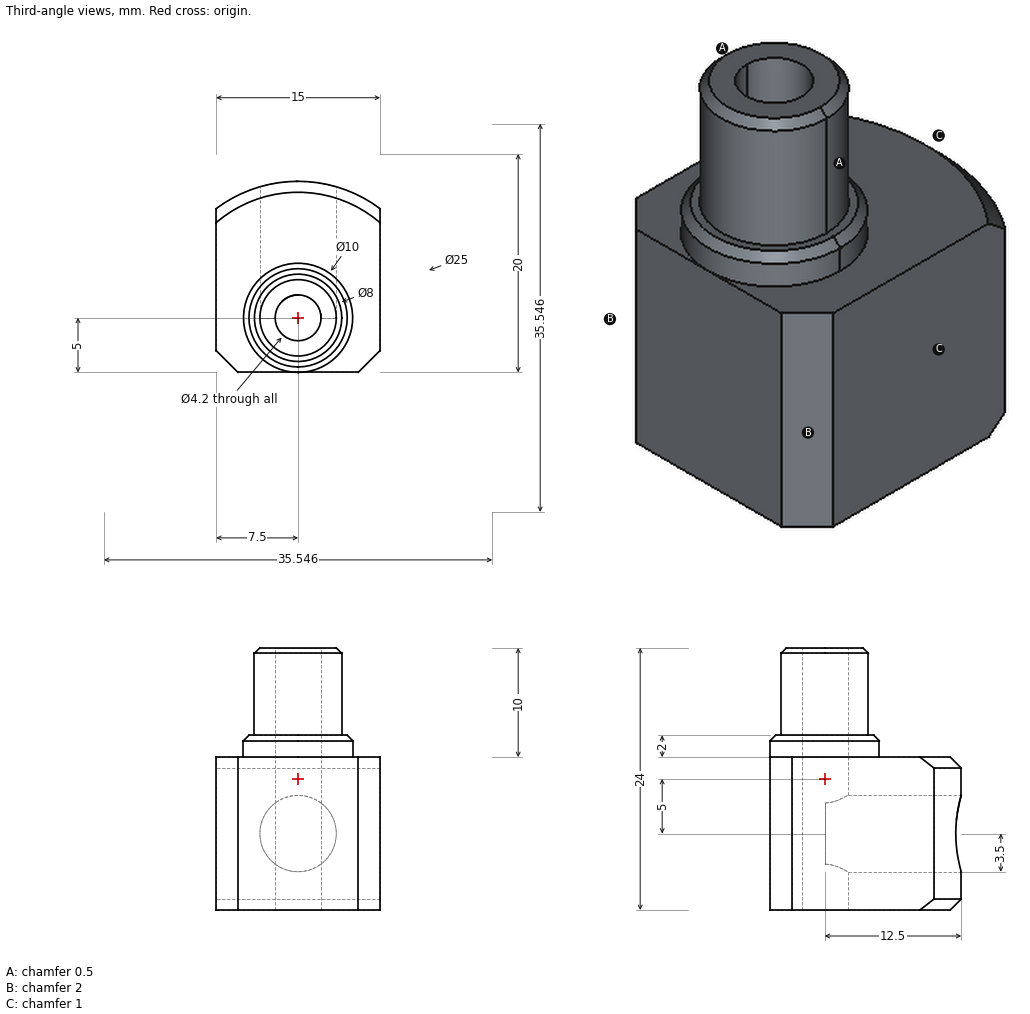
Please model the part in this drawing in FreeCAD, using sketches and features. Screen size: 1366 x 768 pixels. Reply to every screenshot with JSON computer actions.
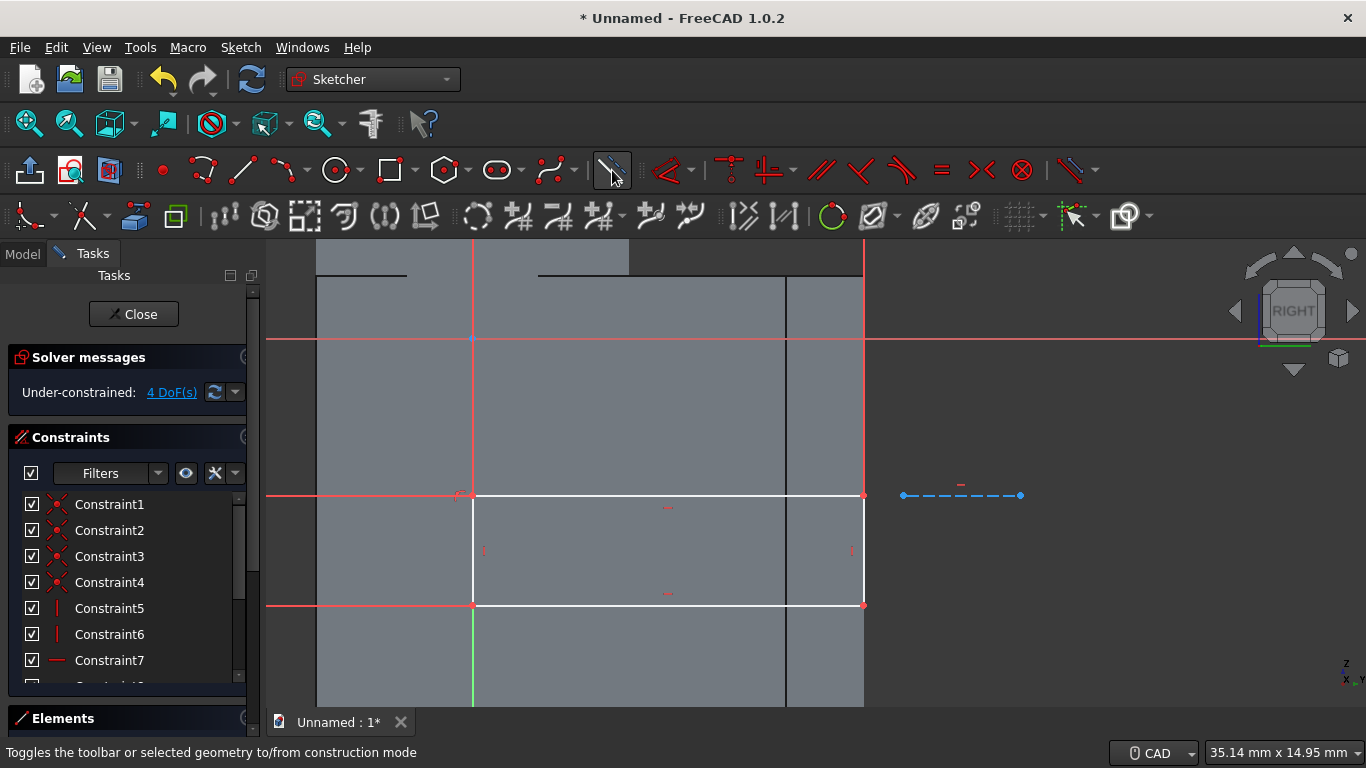
{"action": "left_click", "coordinate": [473, 496]}
{"action": "left_click", "coordinate": [439, 417]}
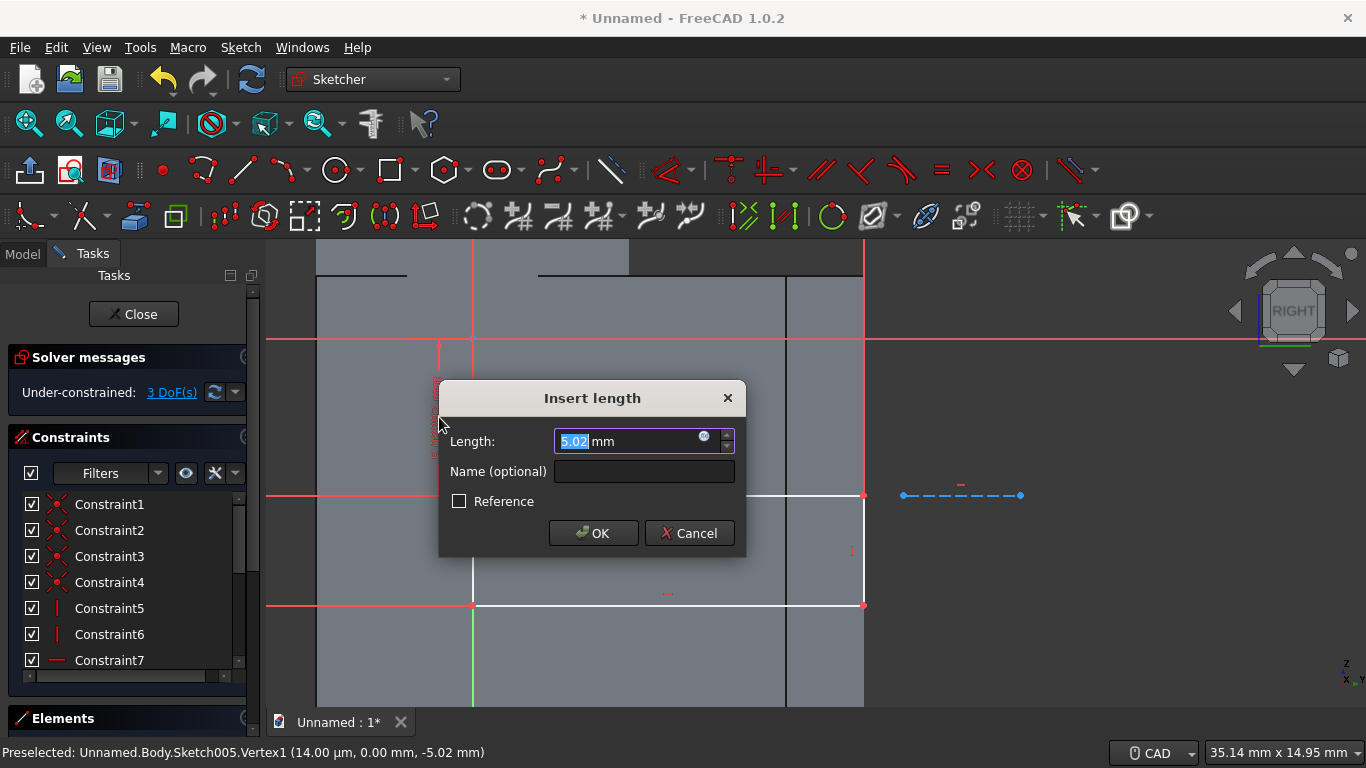
{"action": "type", "text": "5"}
{"action": "key", "text": "Return"}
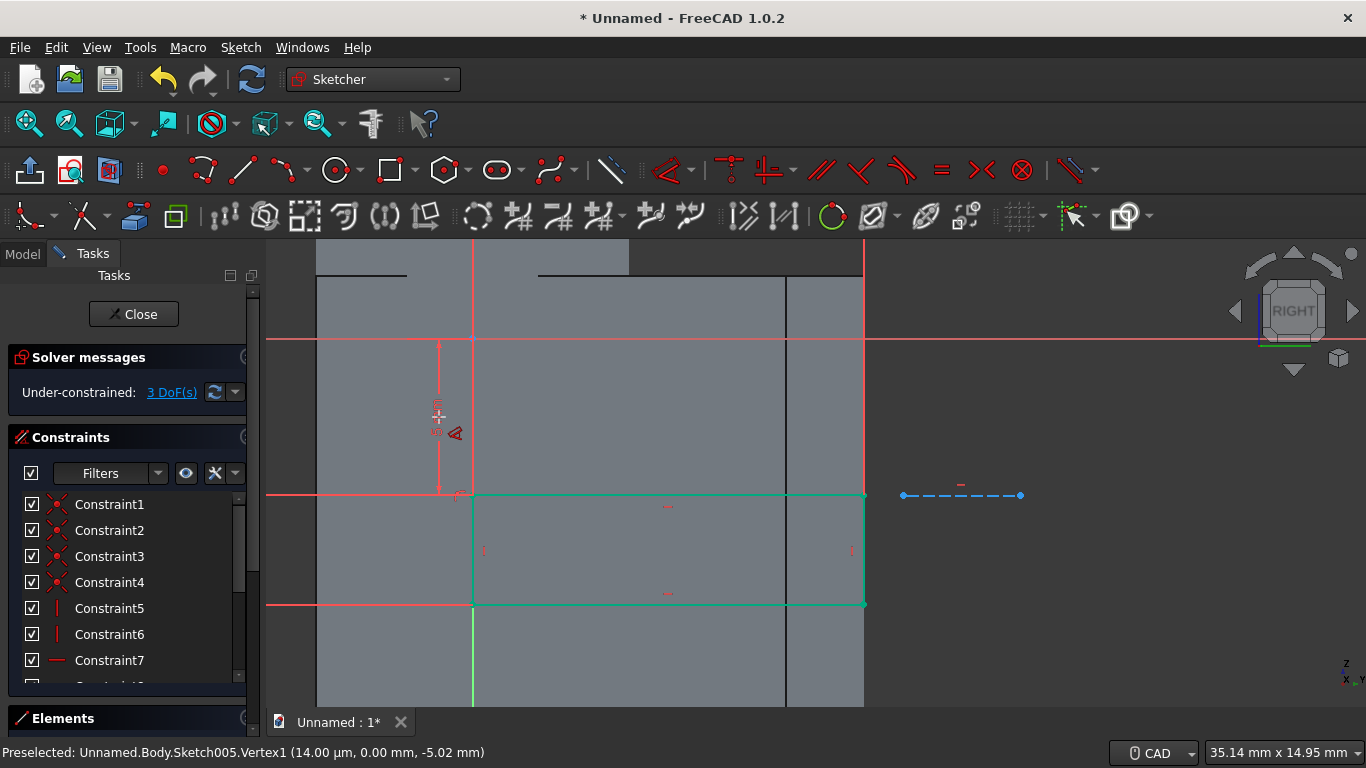
{"action": "left_click", "coordinate": [903, 496]}
{"action": "left_click", "coordinate": [439, 381]}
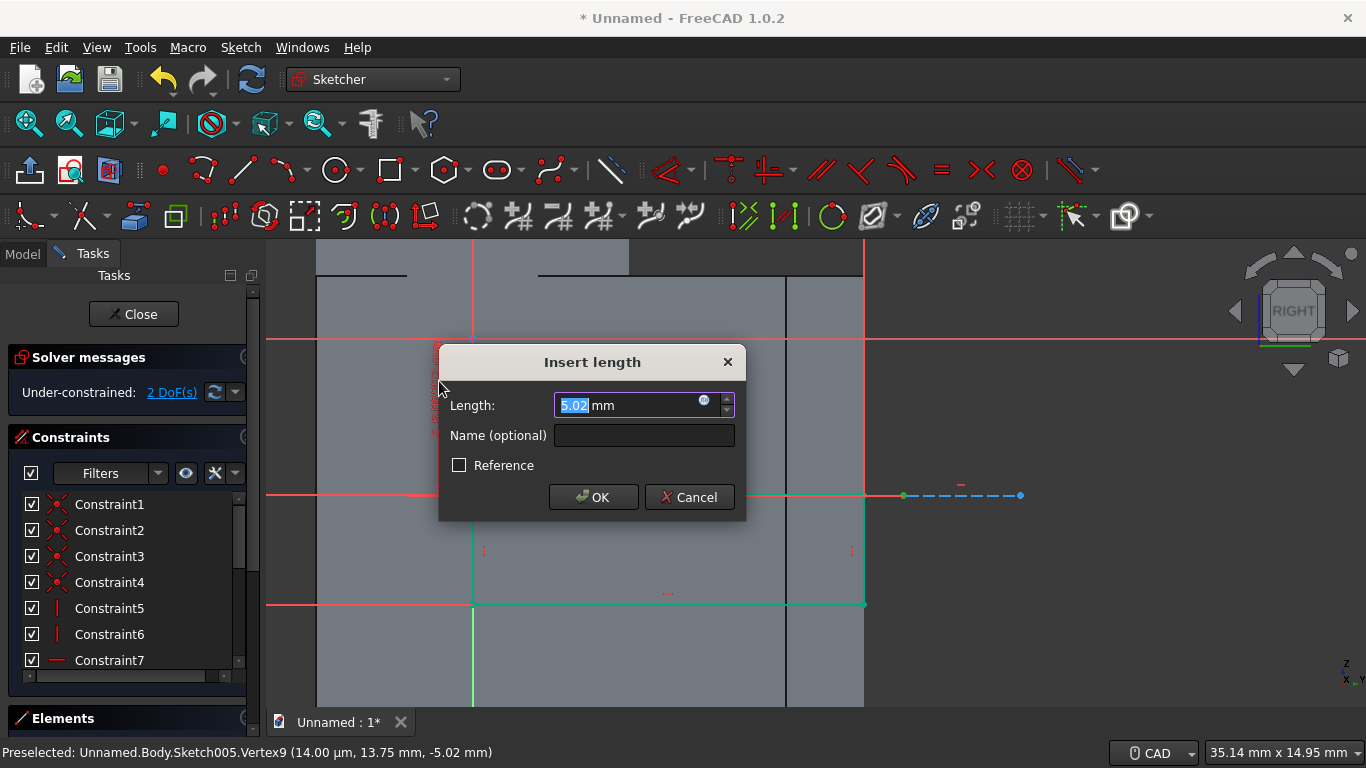
{"action": "type", "text": "5"}
{"action": "key", "text": "Return"}
{"action": "key", "text": "Escape"}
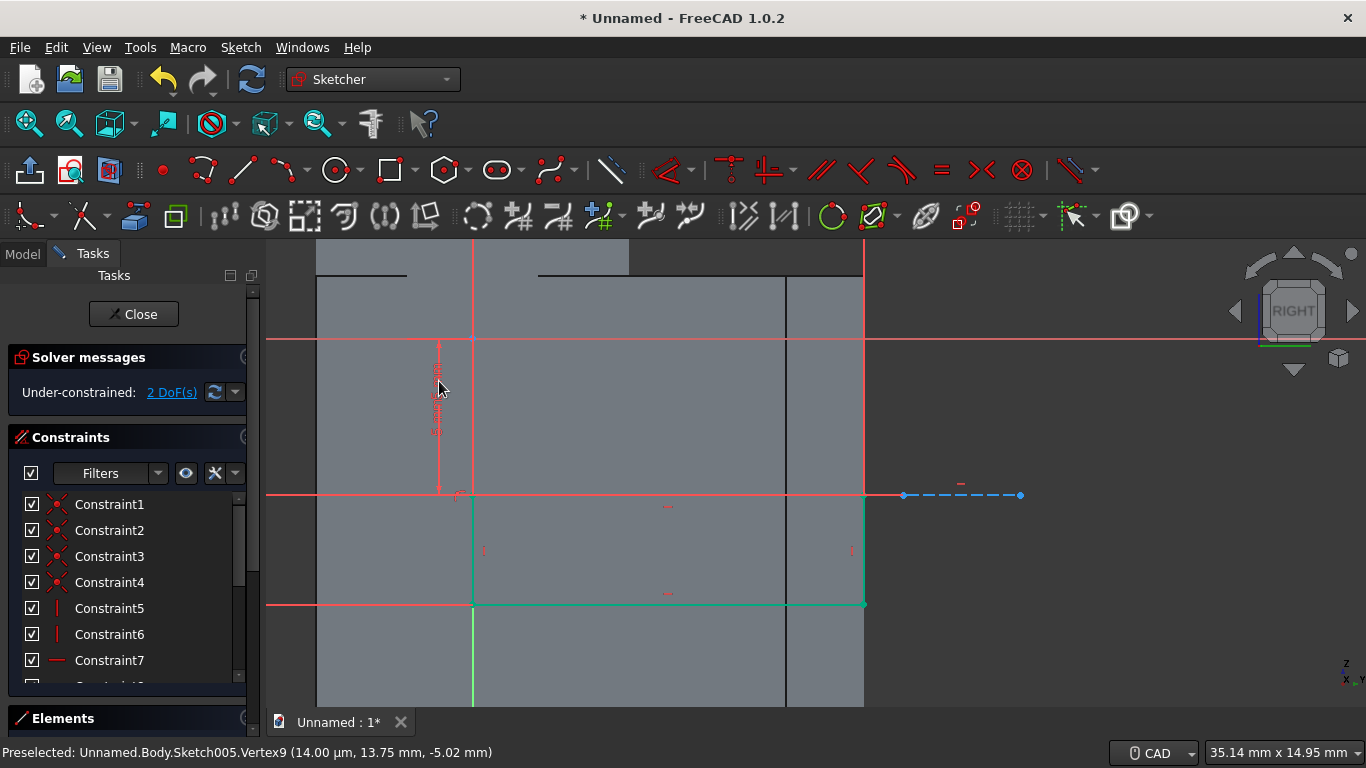
{"action": "left_click", "coordinate": [134, 314]}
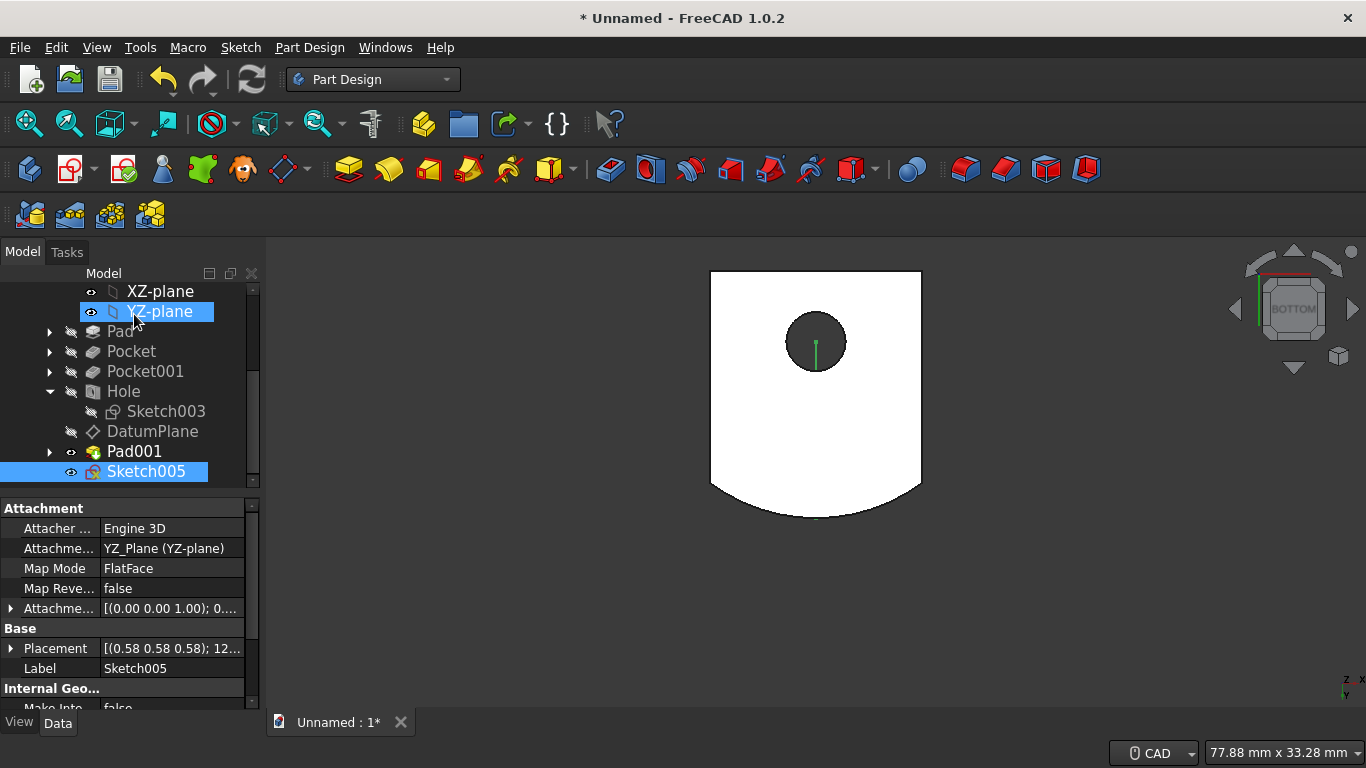
{"action": "left_click", "coordinate": [692, 170]}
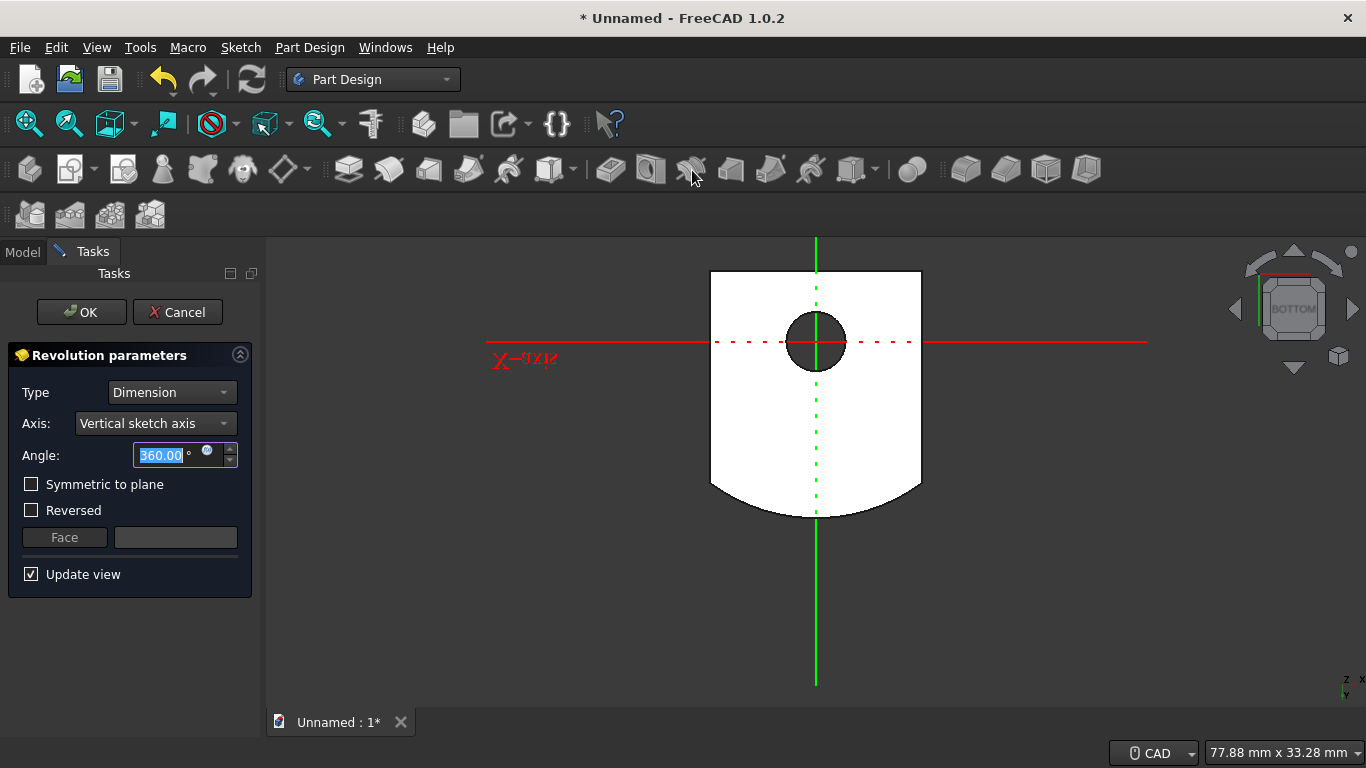
{"action": "left_click", "coordinate": [156, 424]}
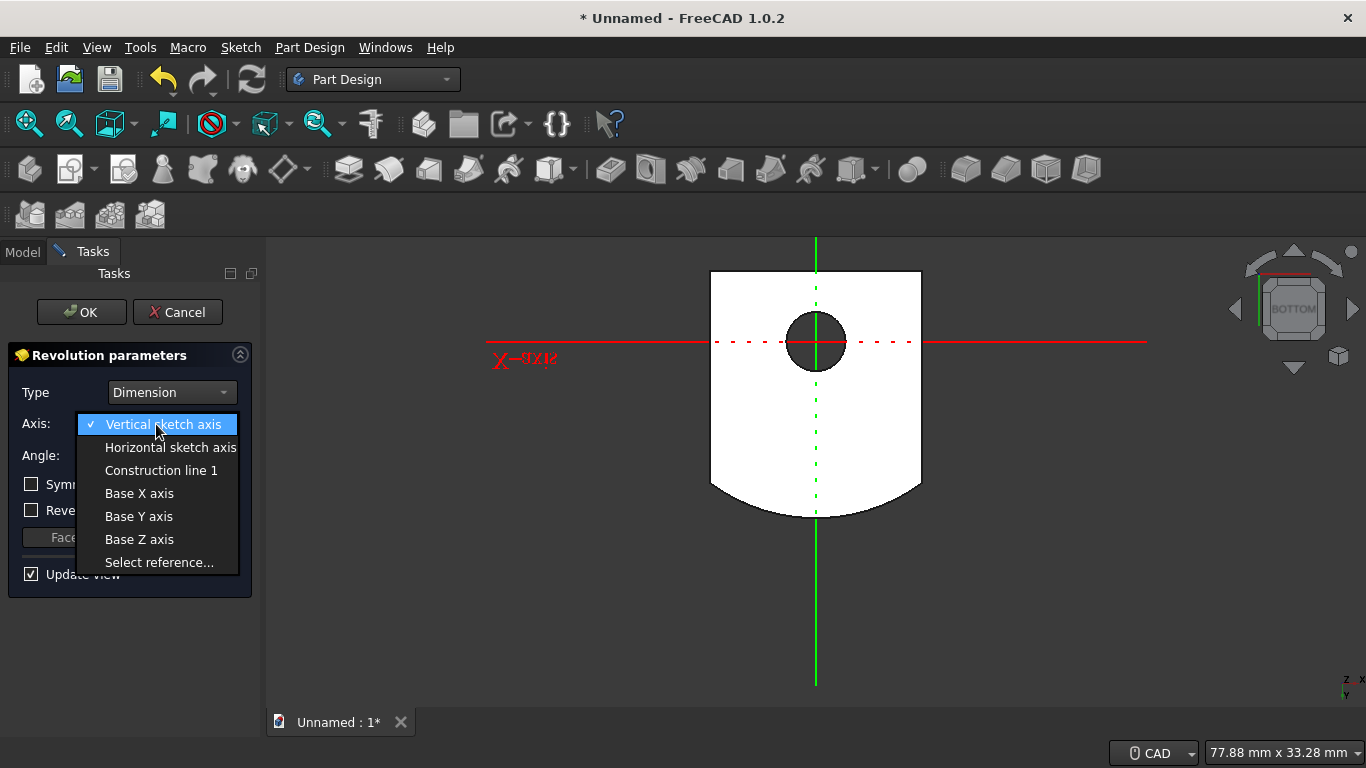
{"action": "left_click", "coordinate": [156, 470]}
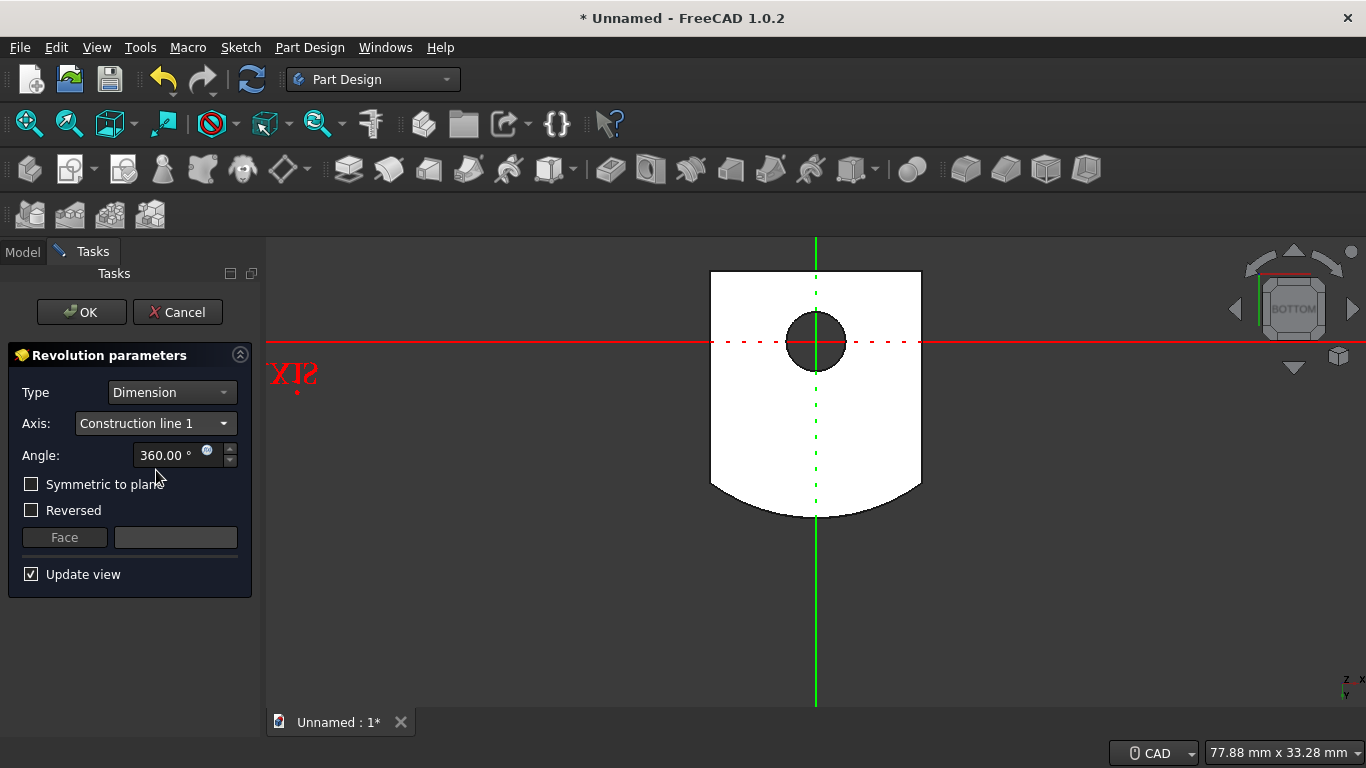
{"action": "left_click", "coordinate": [82, 312]}